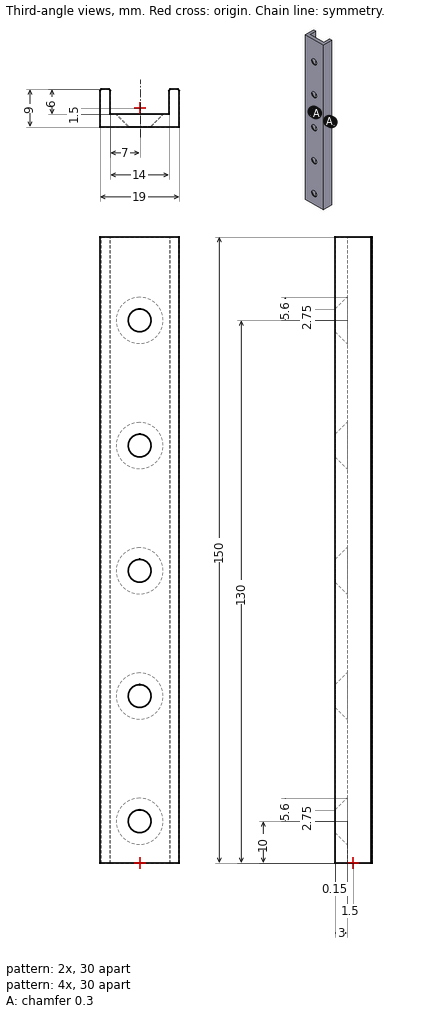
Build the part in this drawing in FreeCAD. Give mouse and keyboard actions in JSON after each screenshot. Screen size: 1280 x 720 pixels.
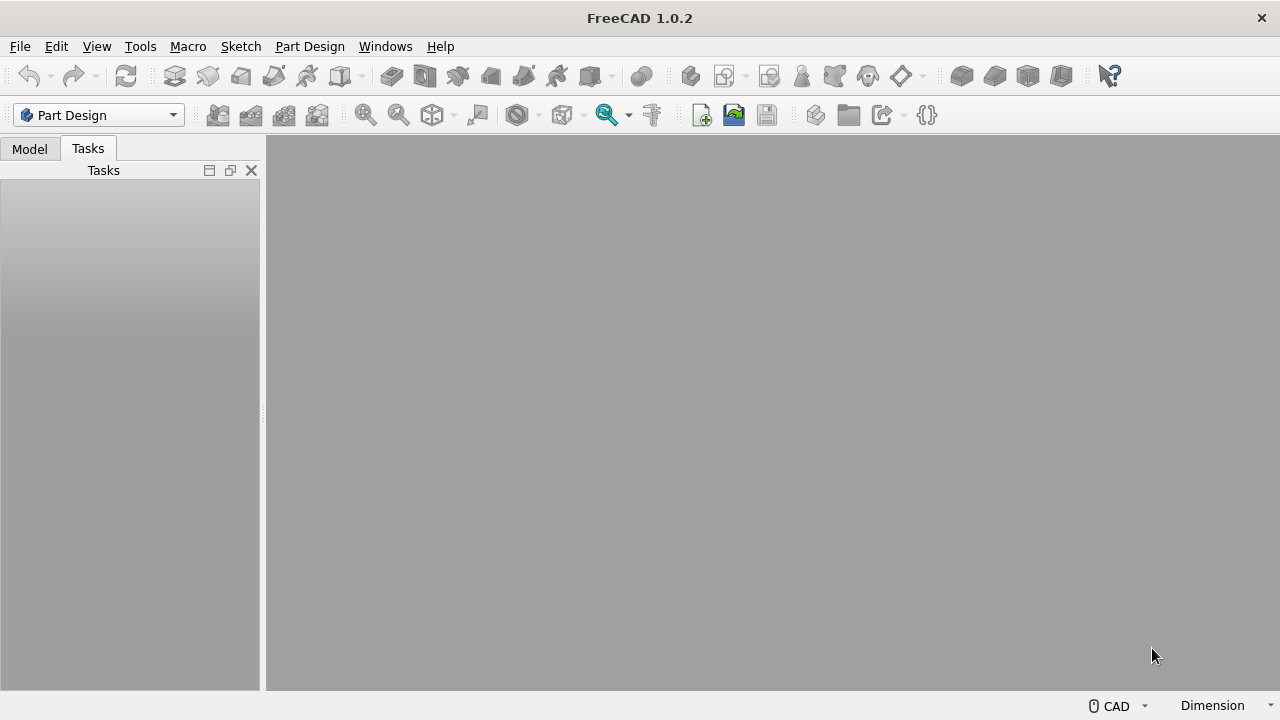
{"action": "key", "text": "ctrl+n"}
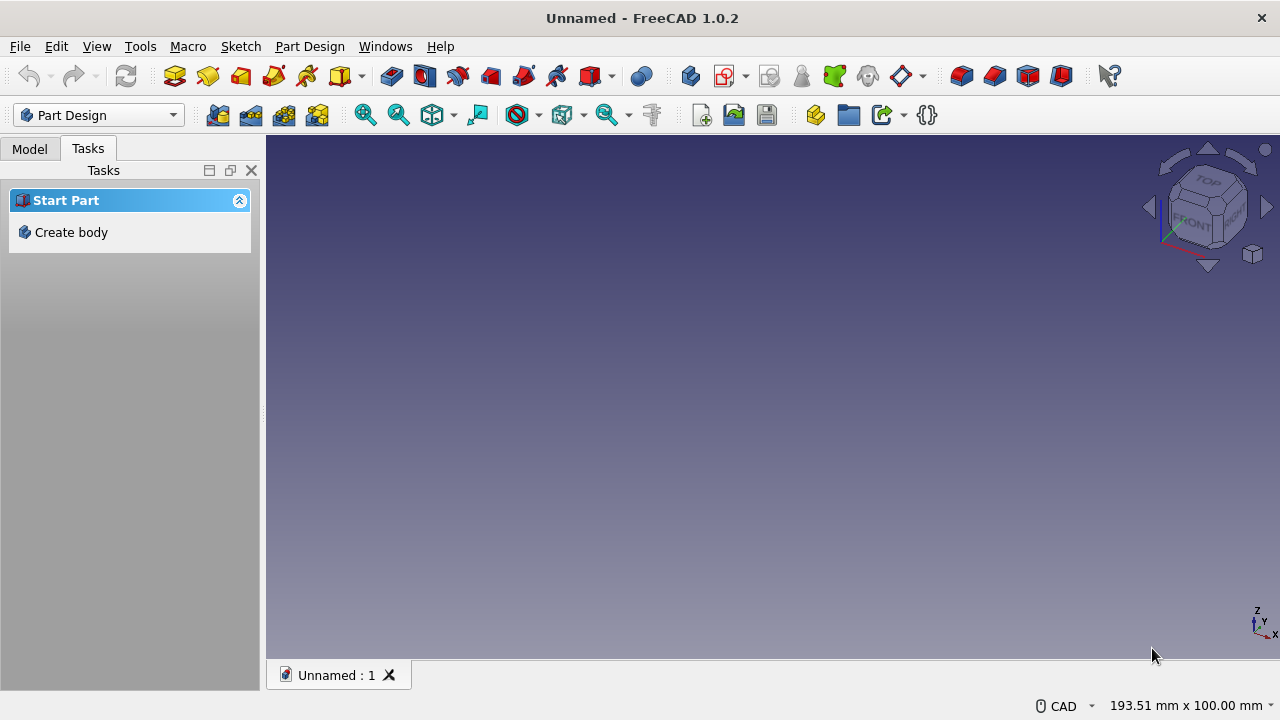
{"action": "left_click", "coordinate": [724, 76]}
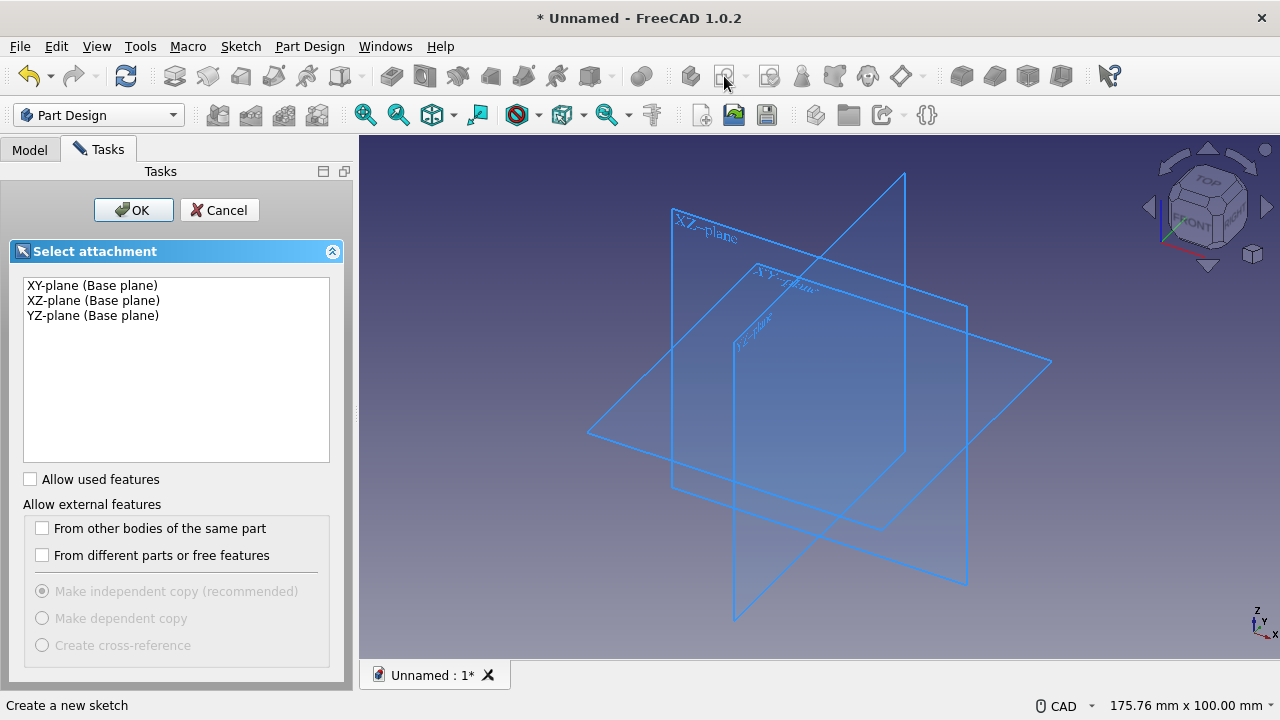
{"action": "left_click", "coordinate": [84, 286]}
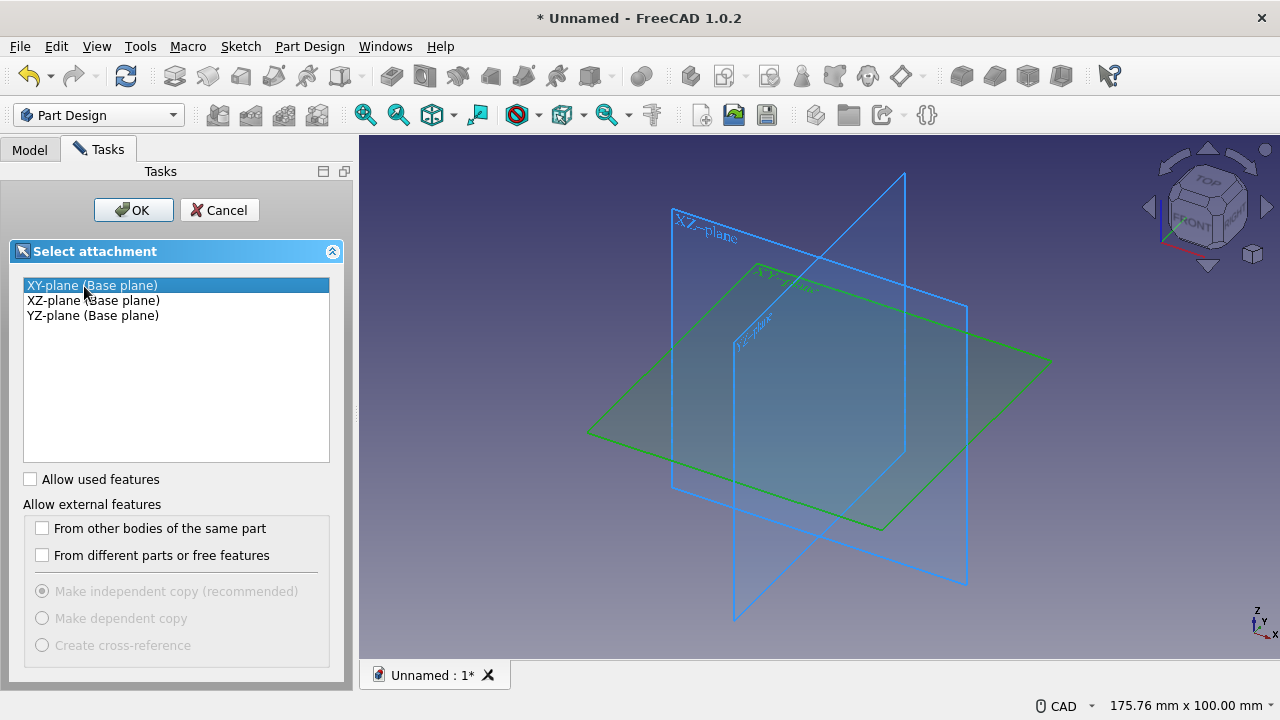
{"action": "left_click", "coordinate": [134, 210]}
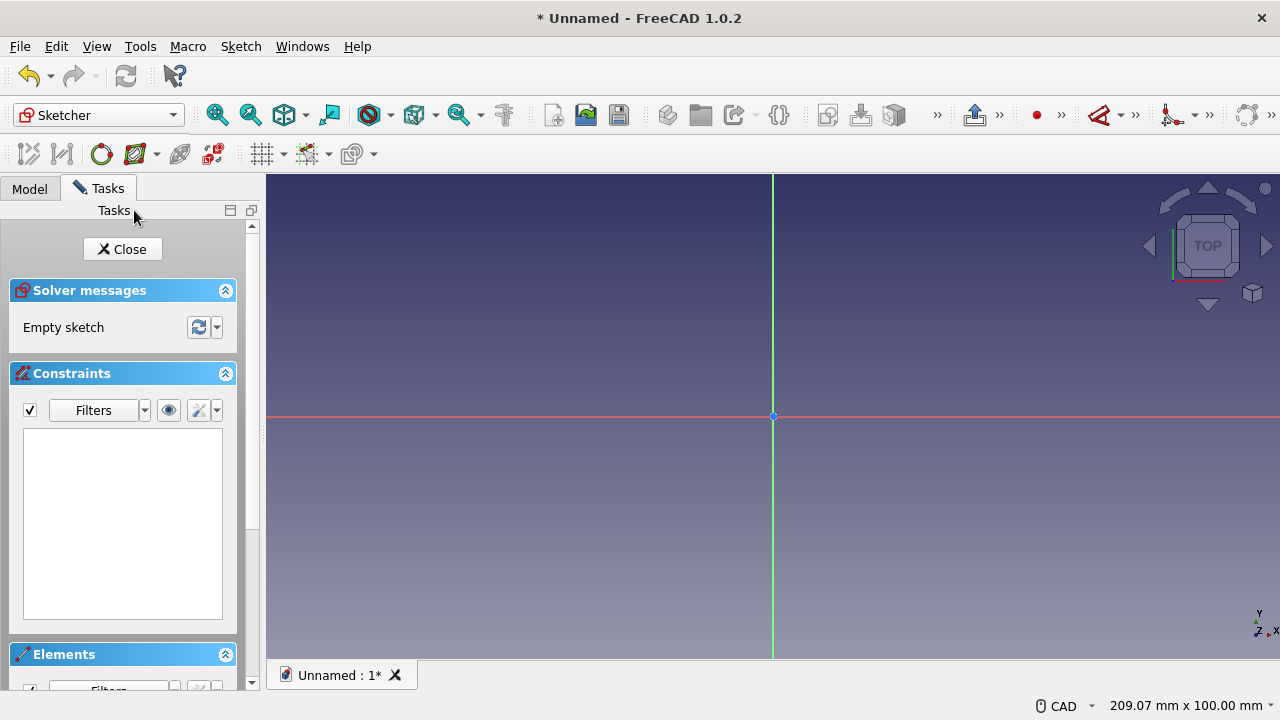
{"action": "scroll", "coordinate": [787, 416], "scroll_direction": "up", "scroll_amount": 9}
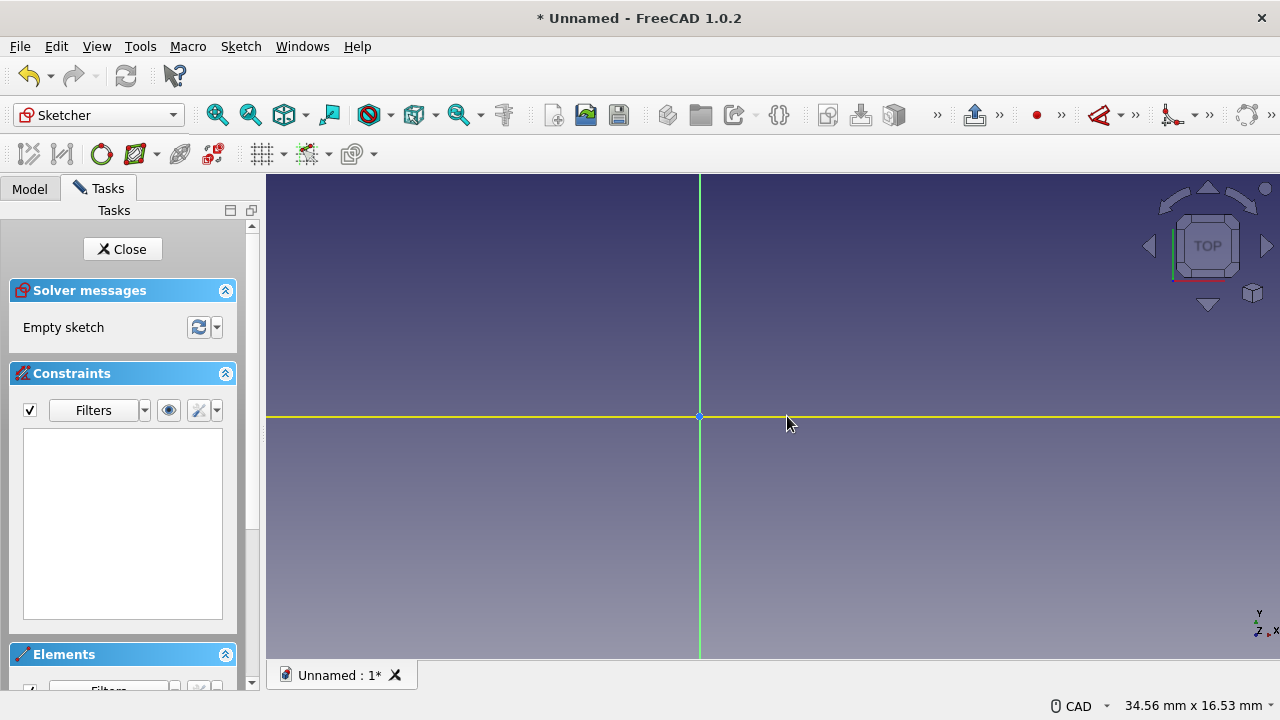
{"action": "key", "text": "g m"}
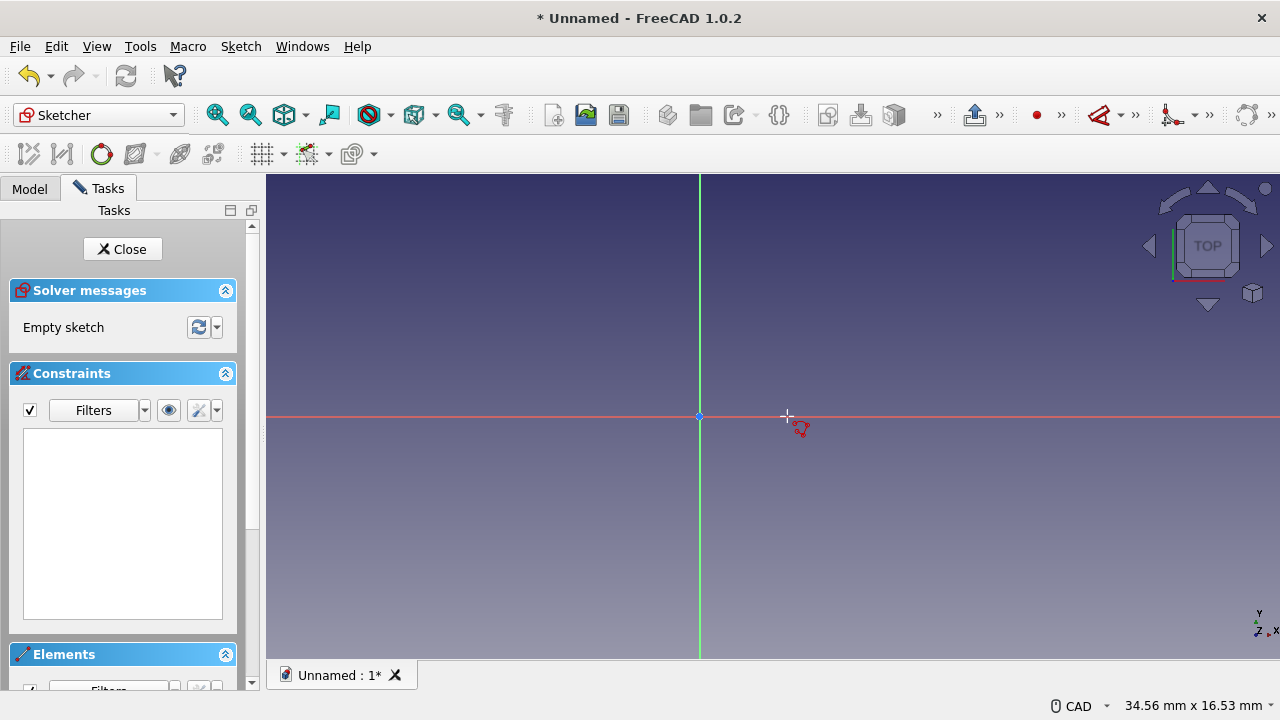
{"action": "left_click", "coordinate": [494, 461]}
{"action": "left_click", "coordinate": [494, 284]}
{"action": "left_click", "coordinate": [421, 284]}
{"action": "left_click", "coordinate": [421, 549]}
{"action": "left_click", "coordinate": [978, 549]}
{"action": "left_click", "coordinate": [978, 284]}
{"action": "left_click", "coordinate": [905, 284]}
{"action": "left_click", "coordinate": [905, 461]}
{"action": "left_click", "coordinate": [494, 462]}
{"action": "key", "text": "Escape"}
{"action": "key", "text": "Escape"}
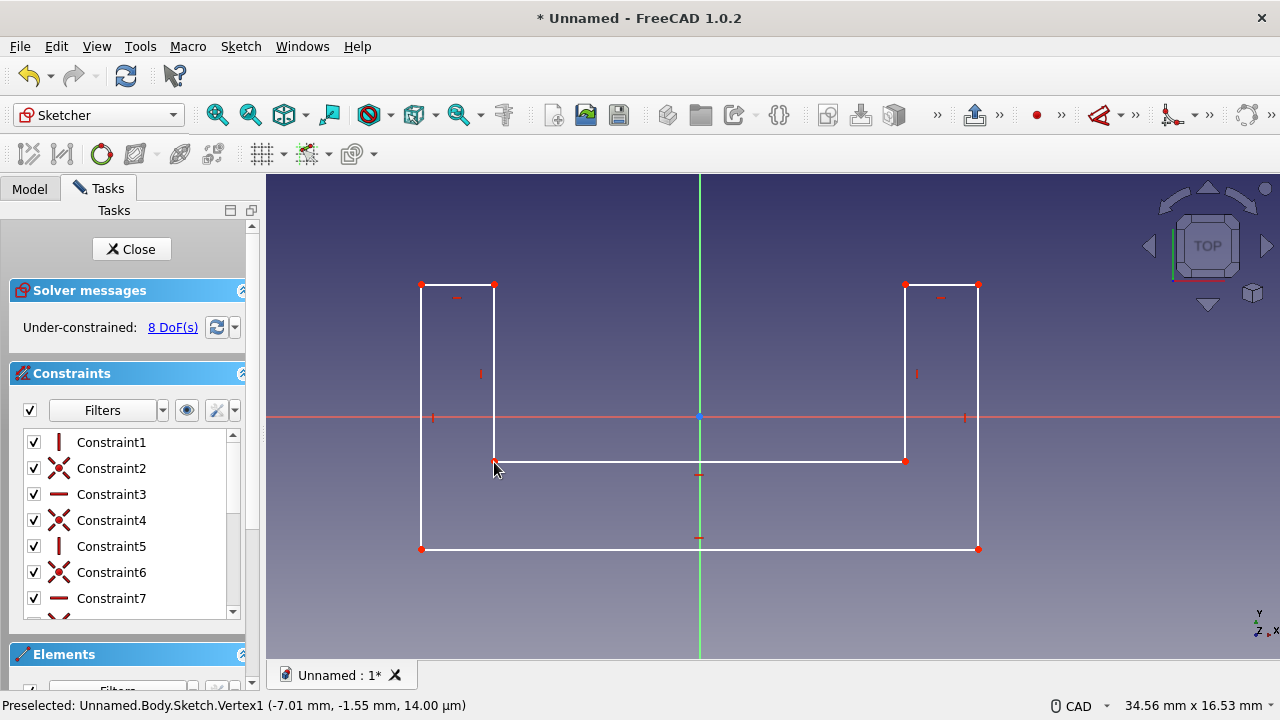
{"action": "left_click", "coordinate": [421, 285]}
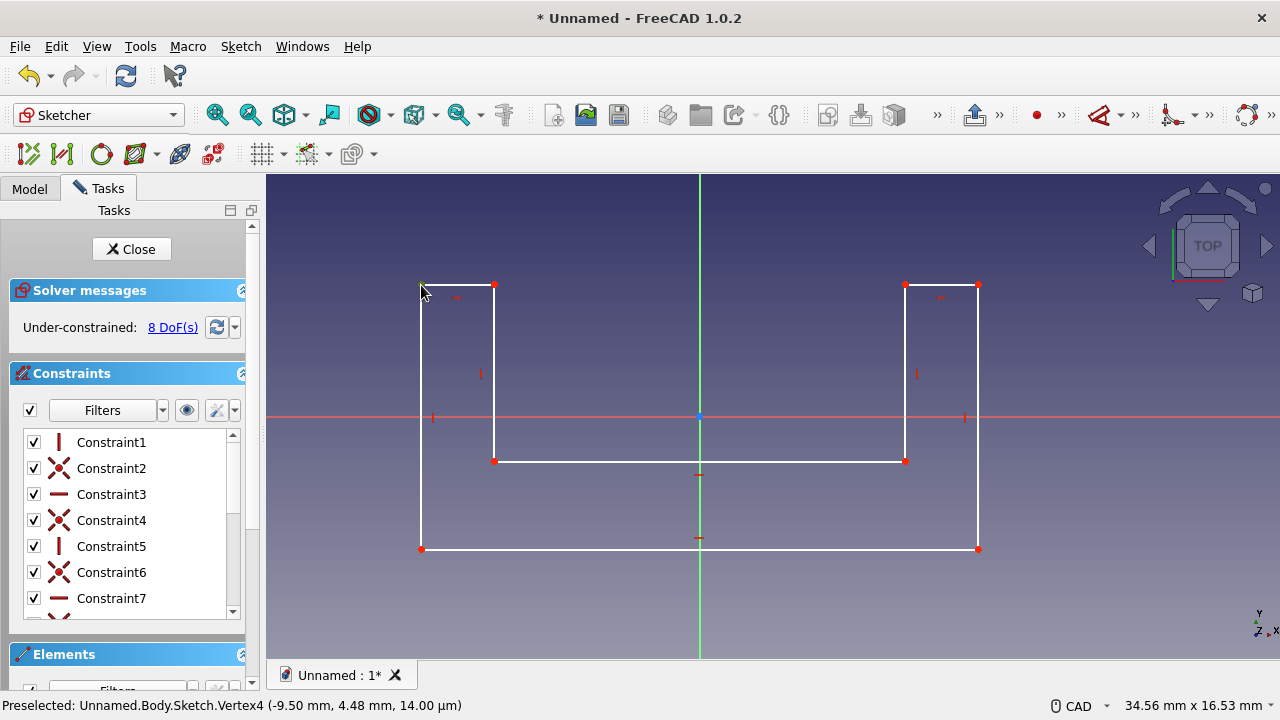
{"action": "left_click", "coordinate": [978, 285]}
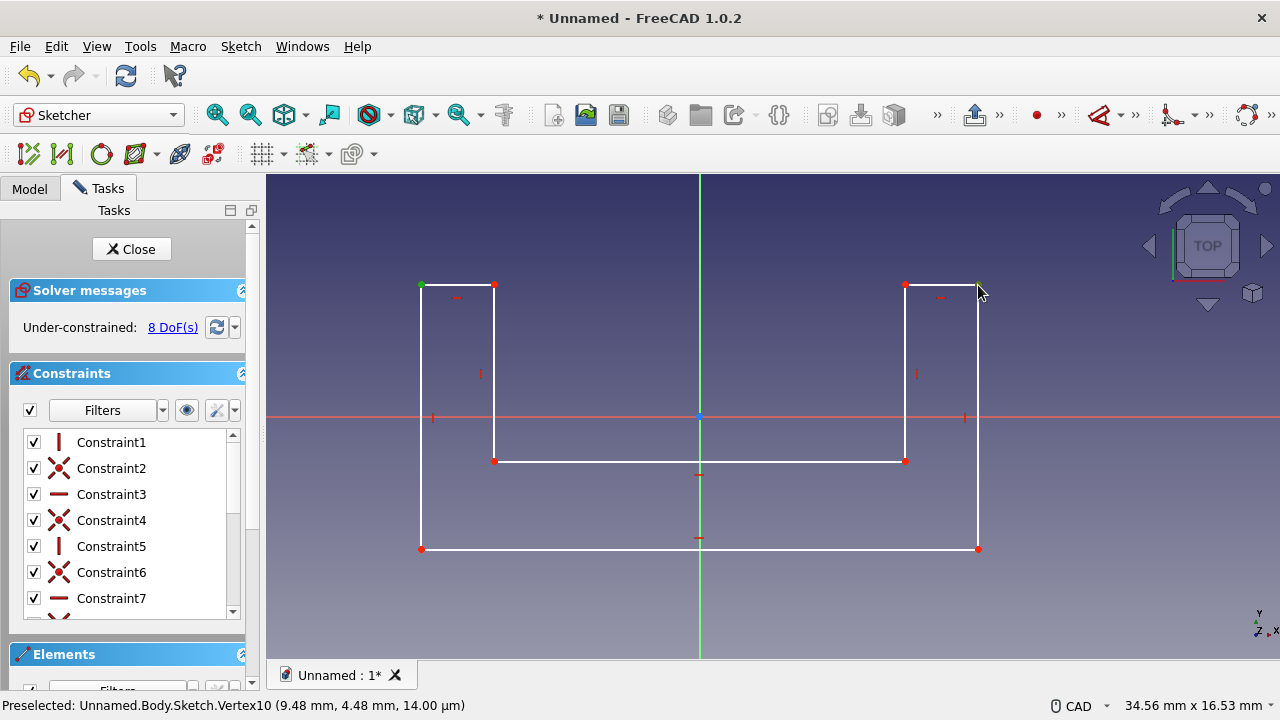
{"action": "left_click", "coordinate": [700, 600]}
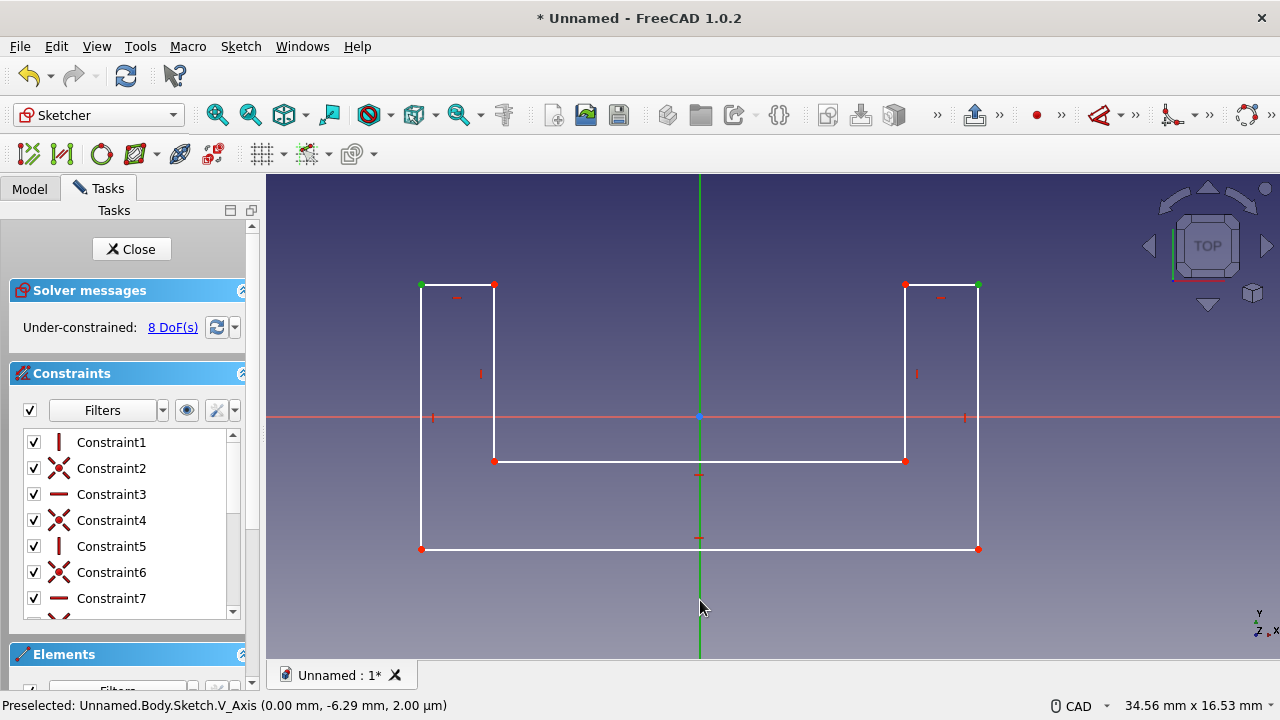
{"action": "key", "text": "s"}